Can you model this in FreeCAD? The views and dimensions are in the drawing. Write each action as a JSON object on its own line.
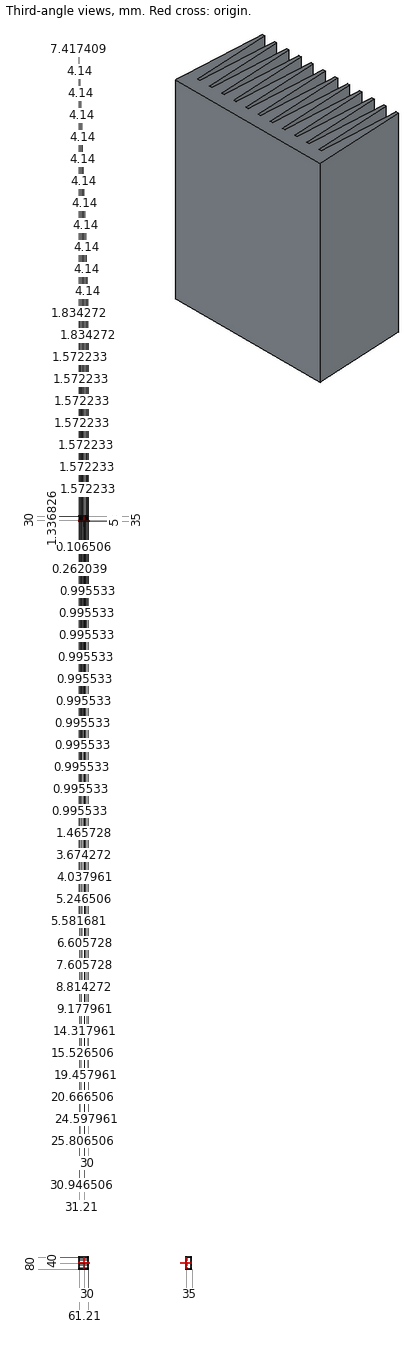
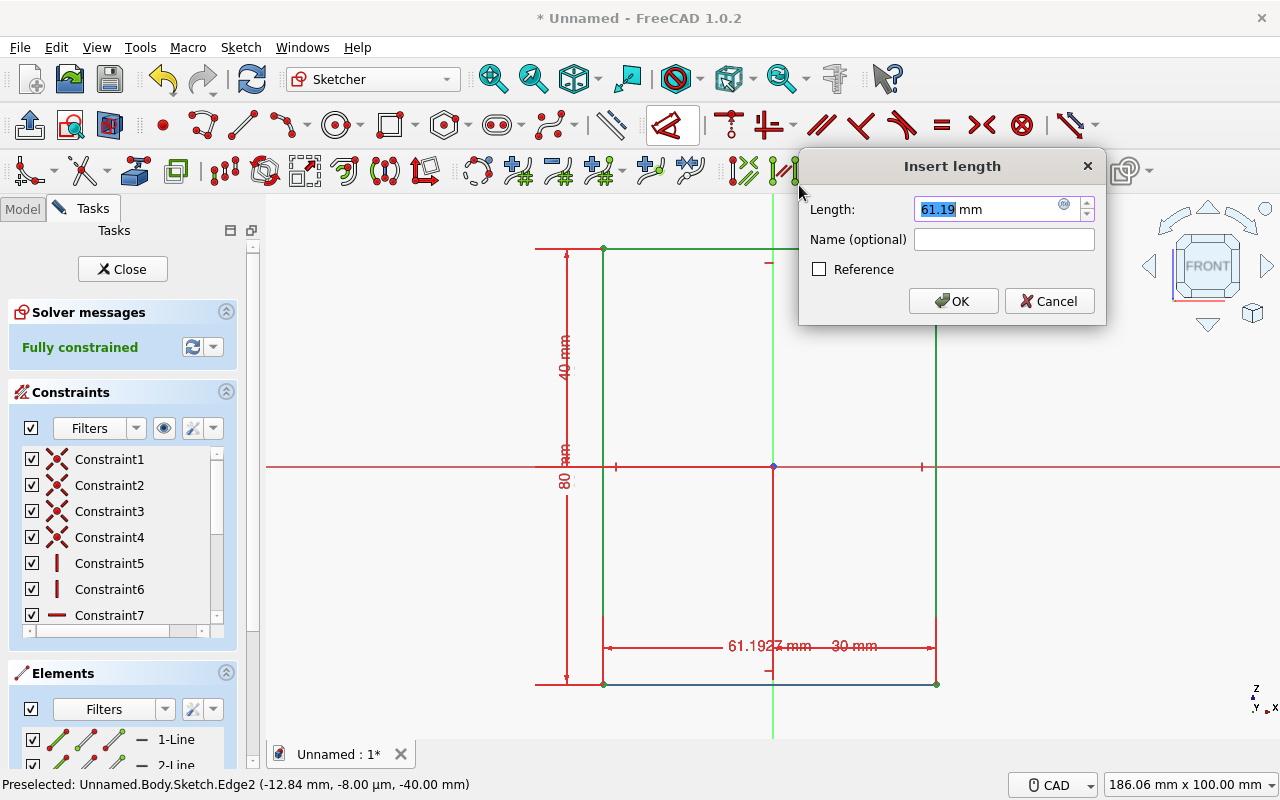
{"action": "type", "text": "61.21"}
{"action": "key", "text": "Return"}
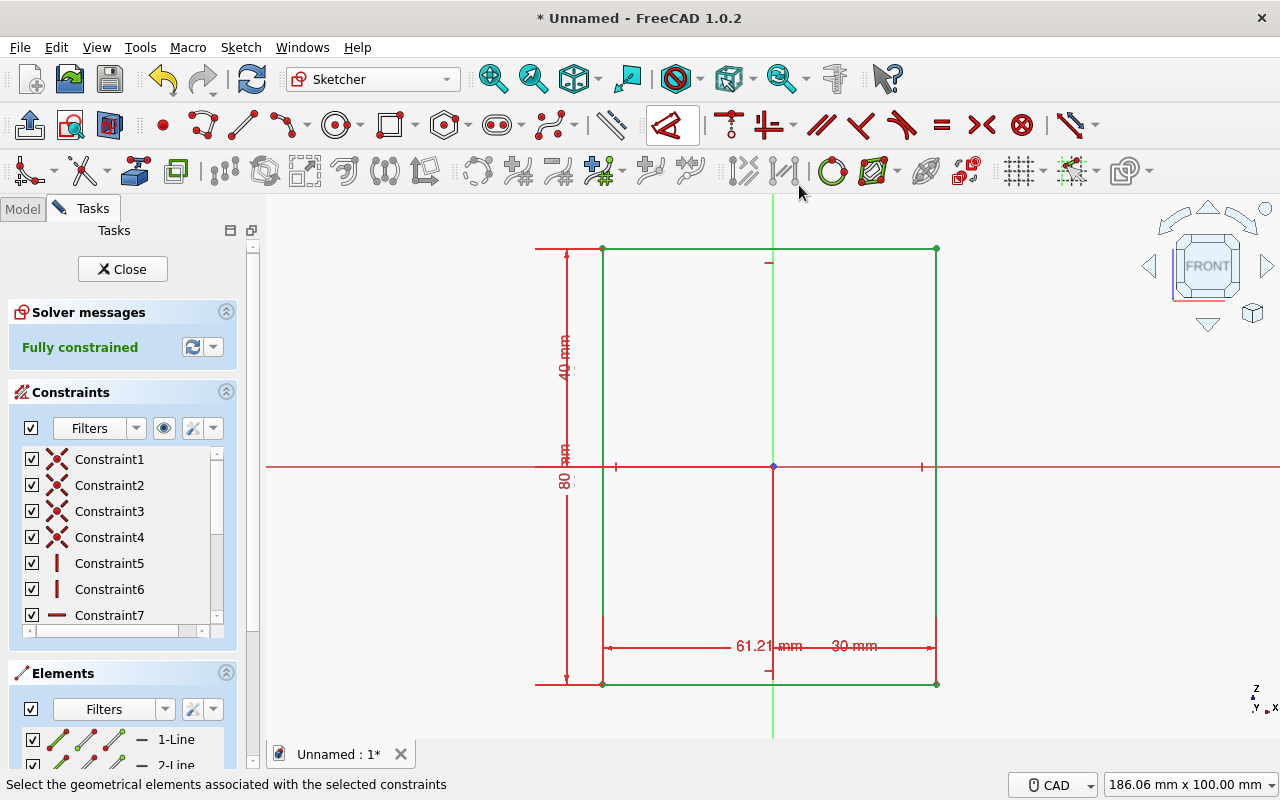
{"action": "left_click", "coordinate": [123, 269]}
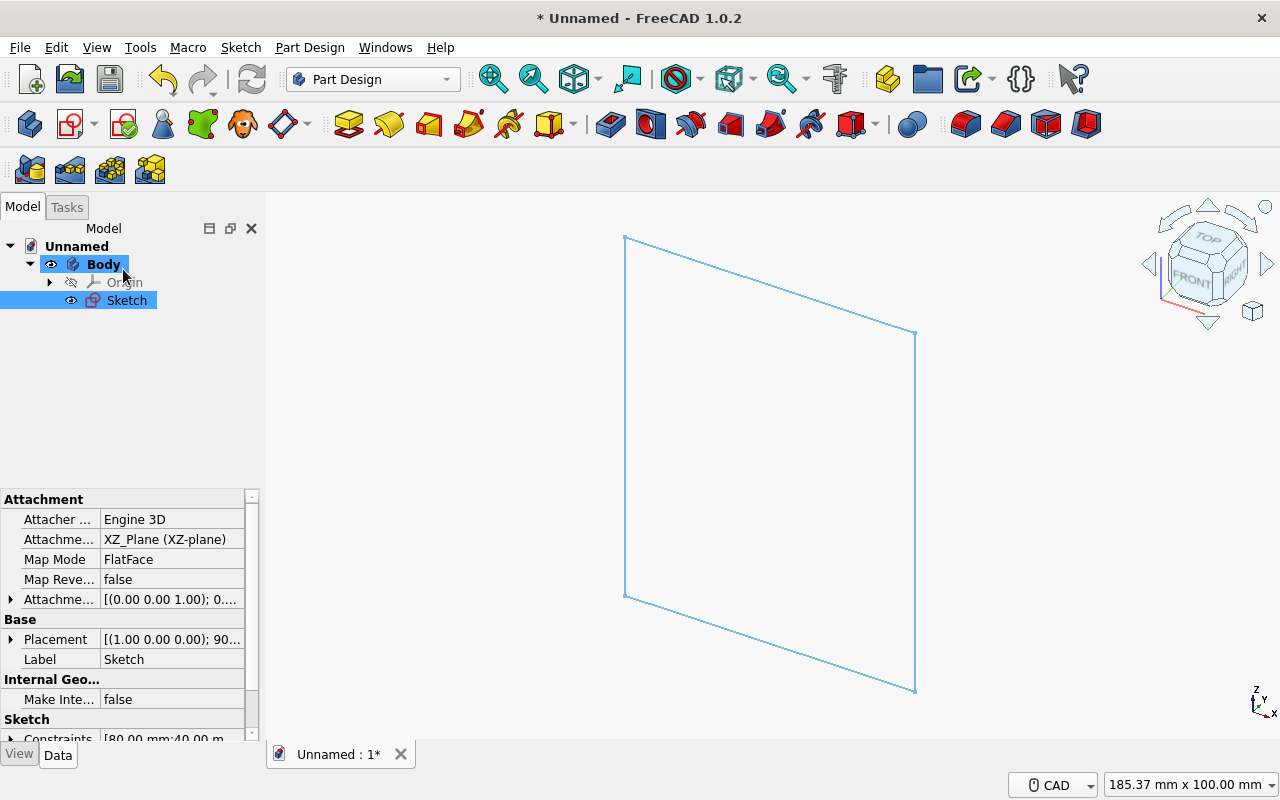
{"action": "left_click", "coordinate": [350, 124]}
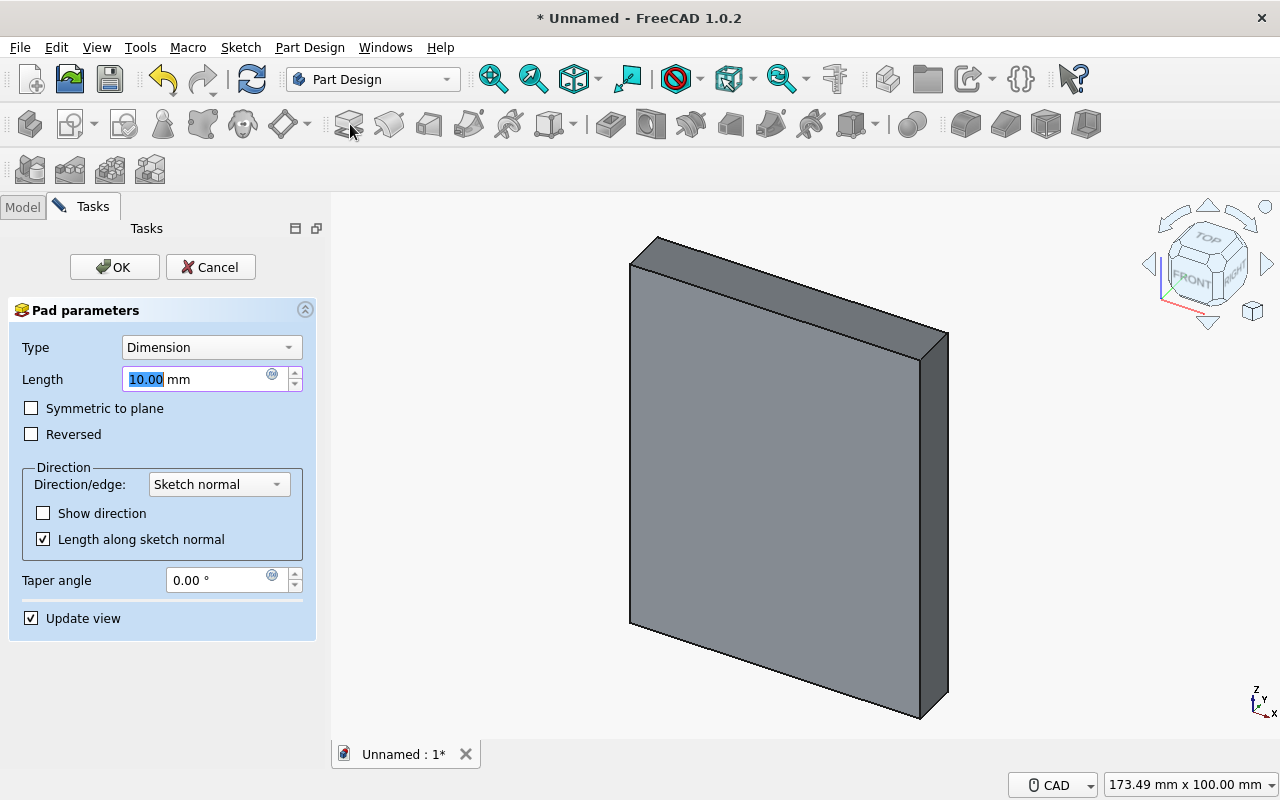
{"action": "type", "text": "35"}
{"action": "key", "text": "Tab"}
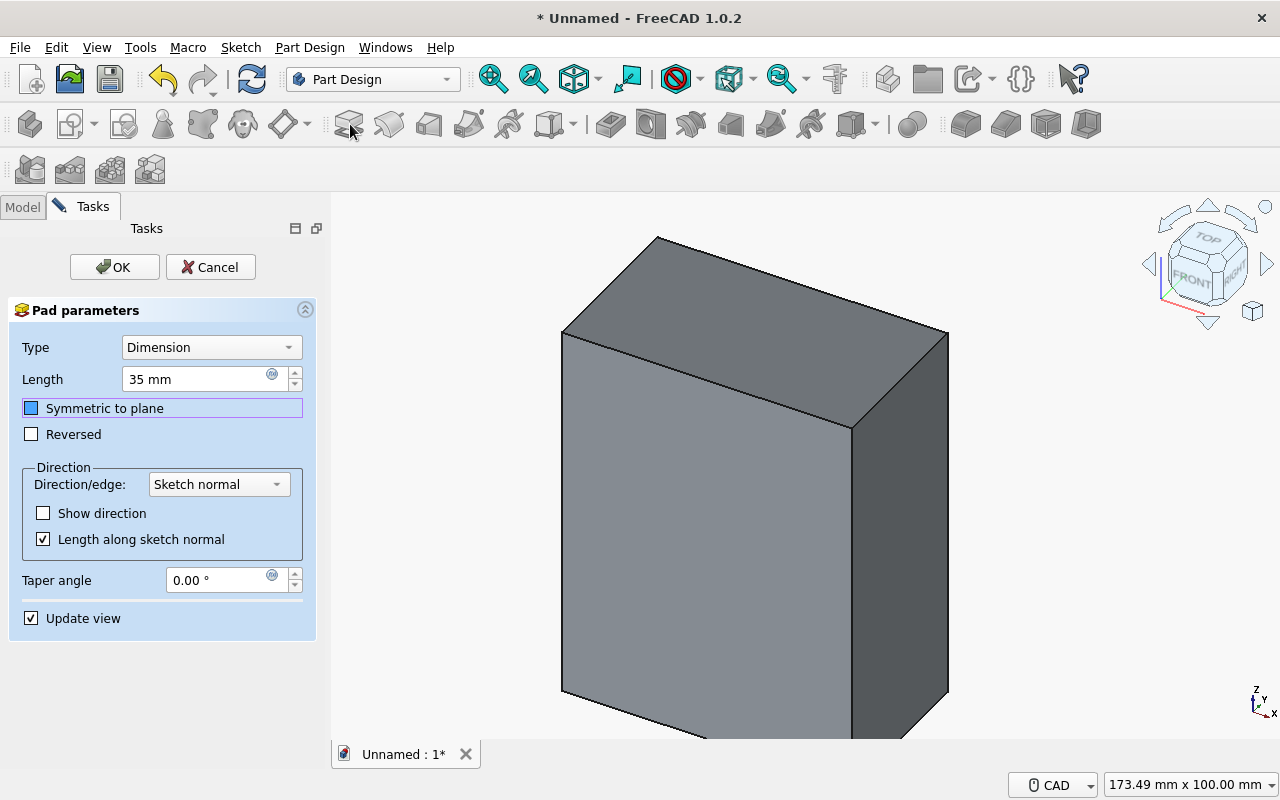
{"action": "left_click", "coordinate": [30, 434]}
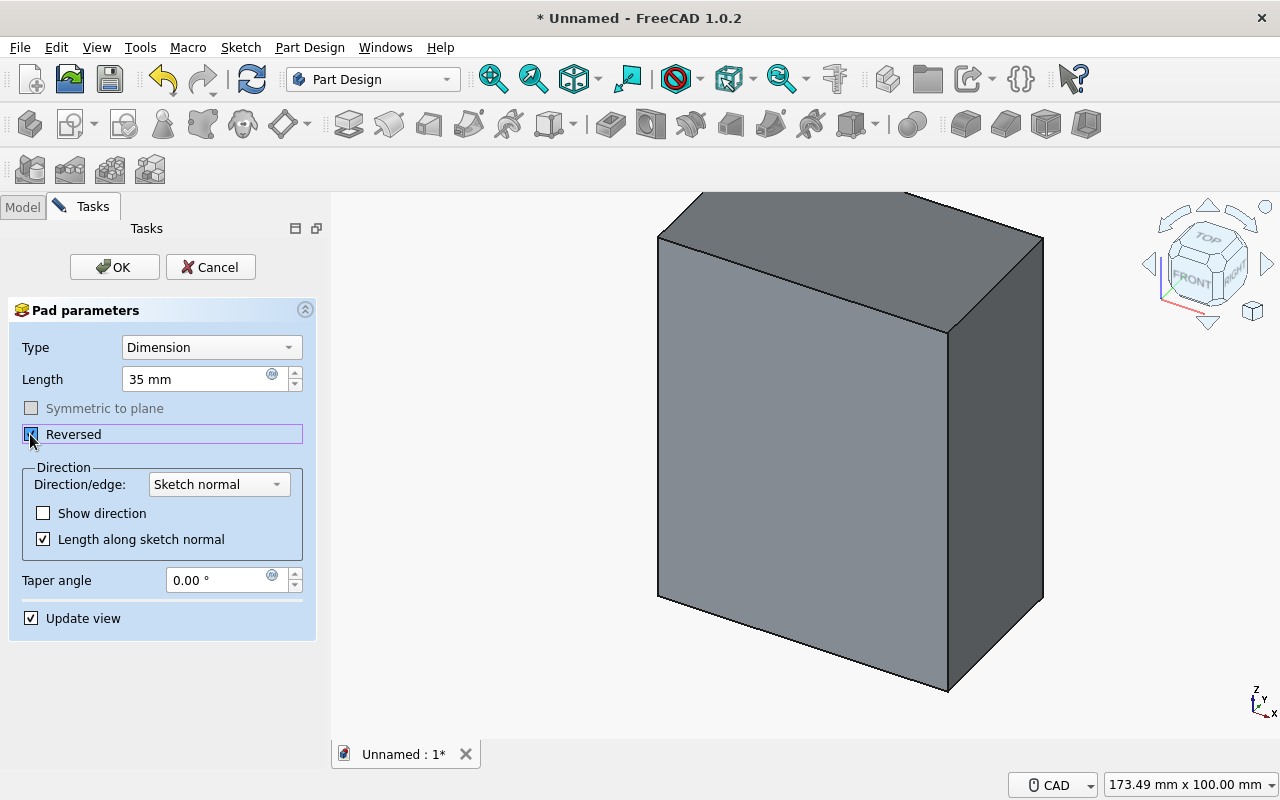
{"action": "left_click", "coordinate": [115, 267]}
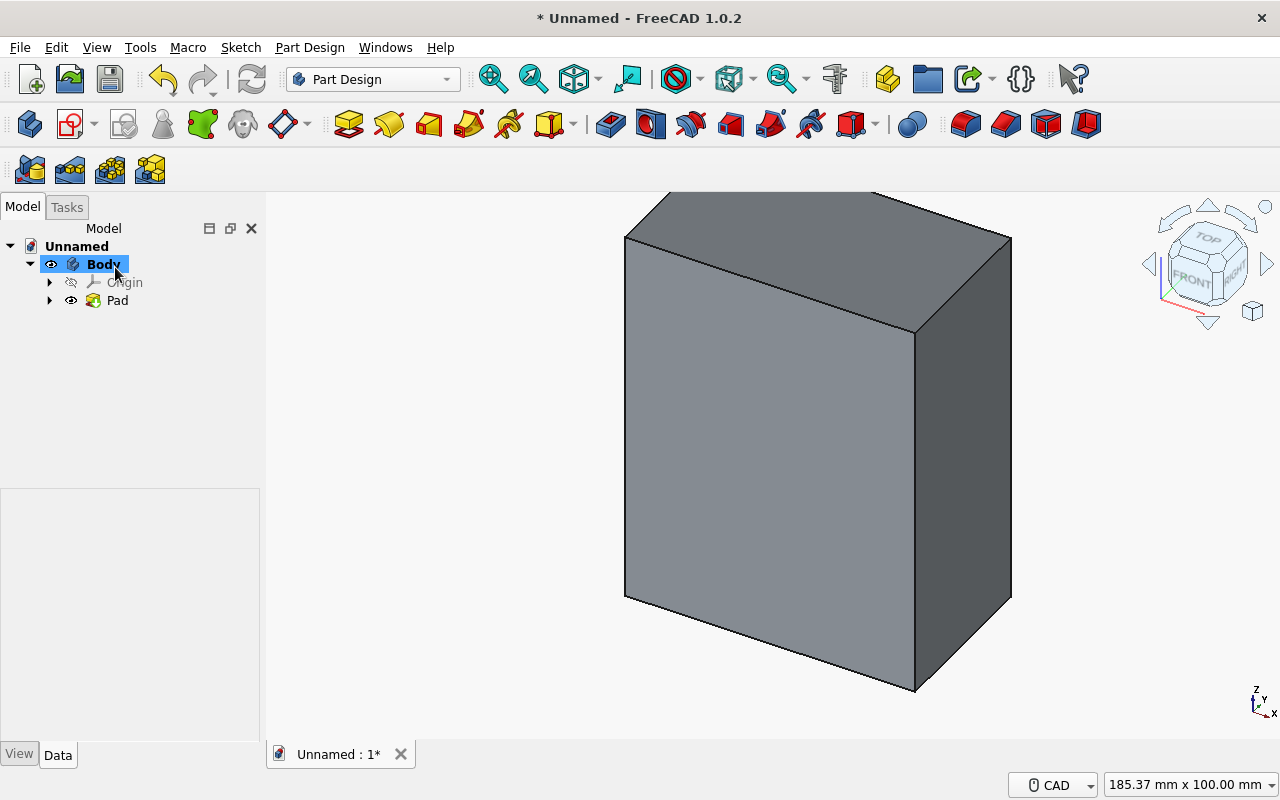
{"action": "left_click", "coordinate": [494, 80]}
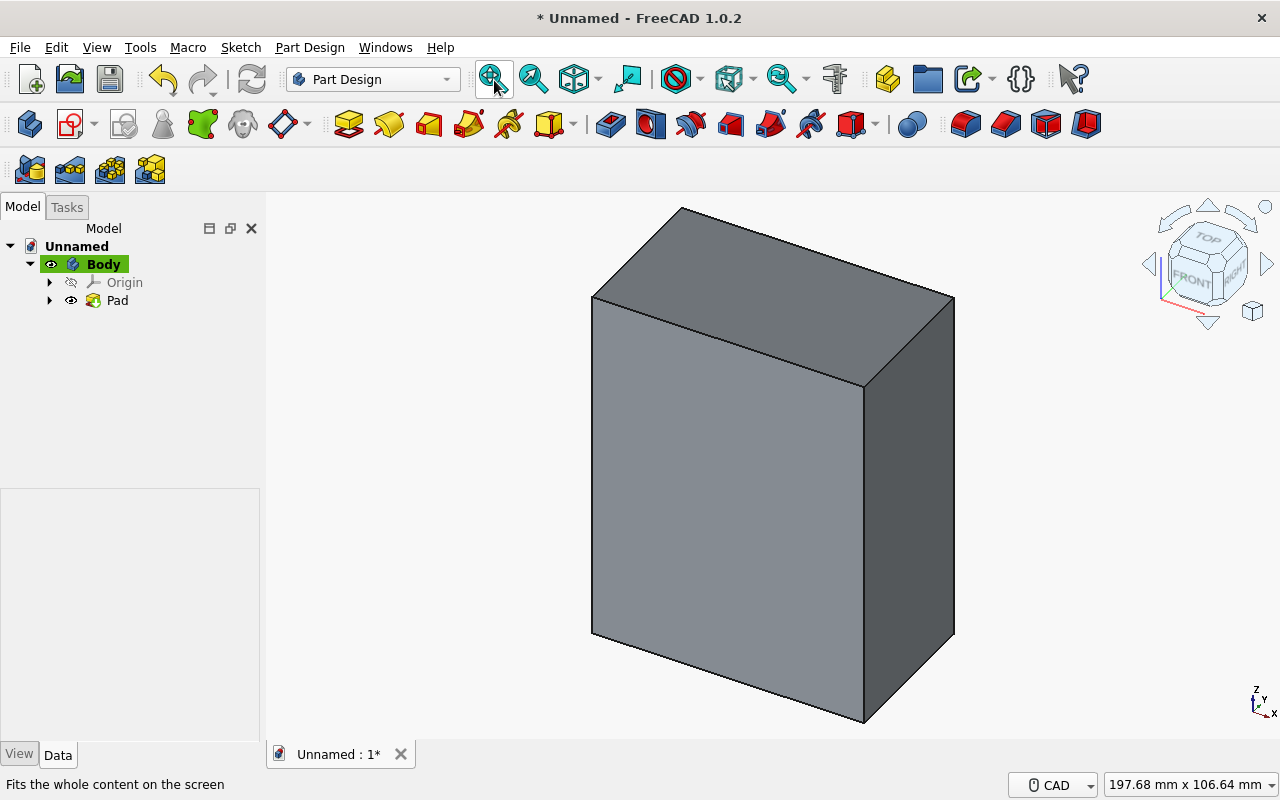
{"action": "left_click", "coordinate": [812, 309]}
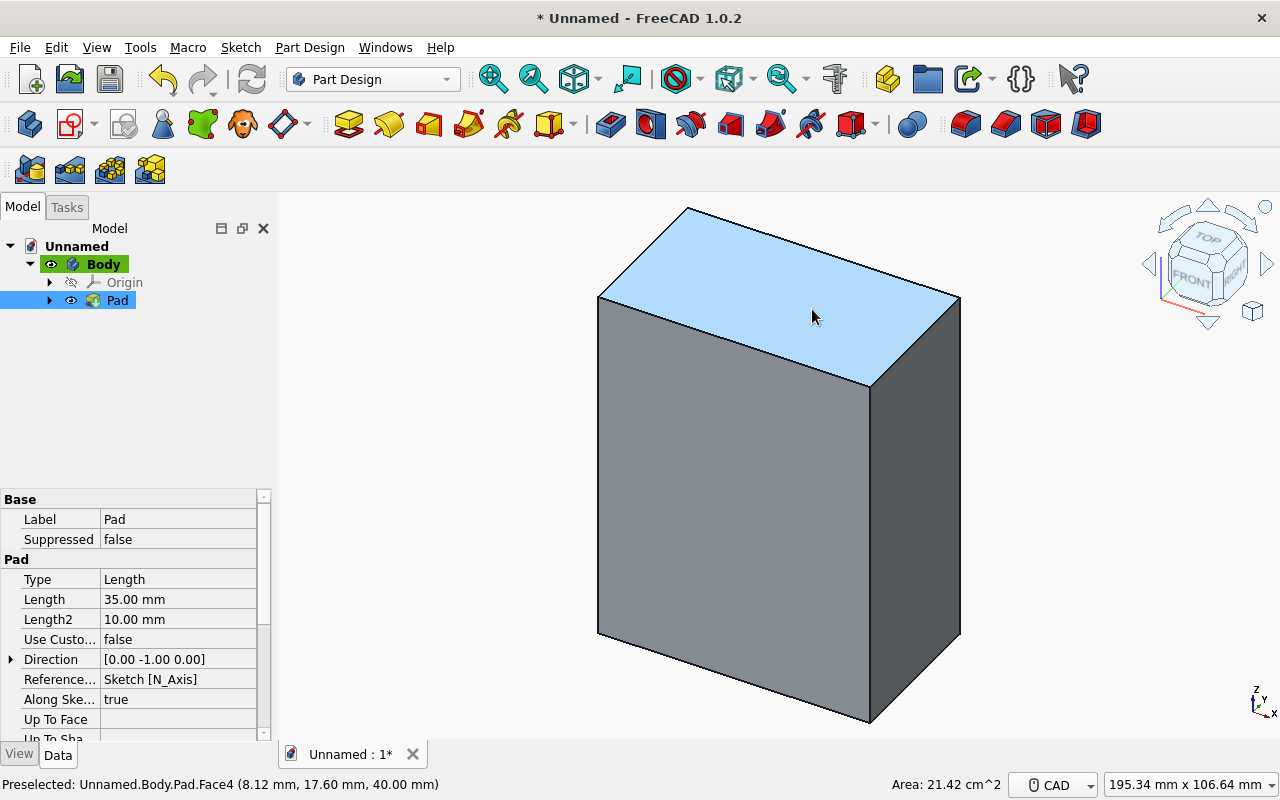
{"action": "left_click", "coordinate": [70, 124]}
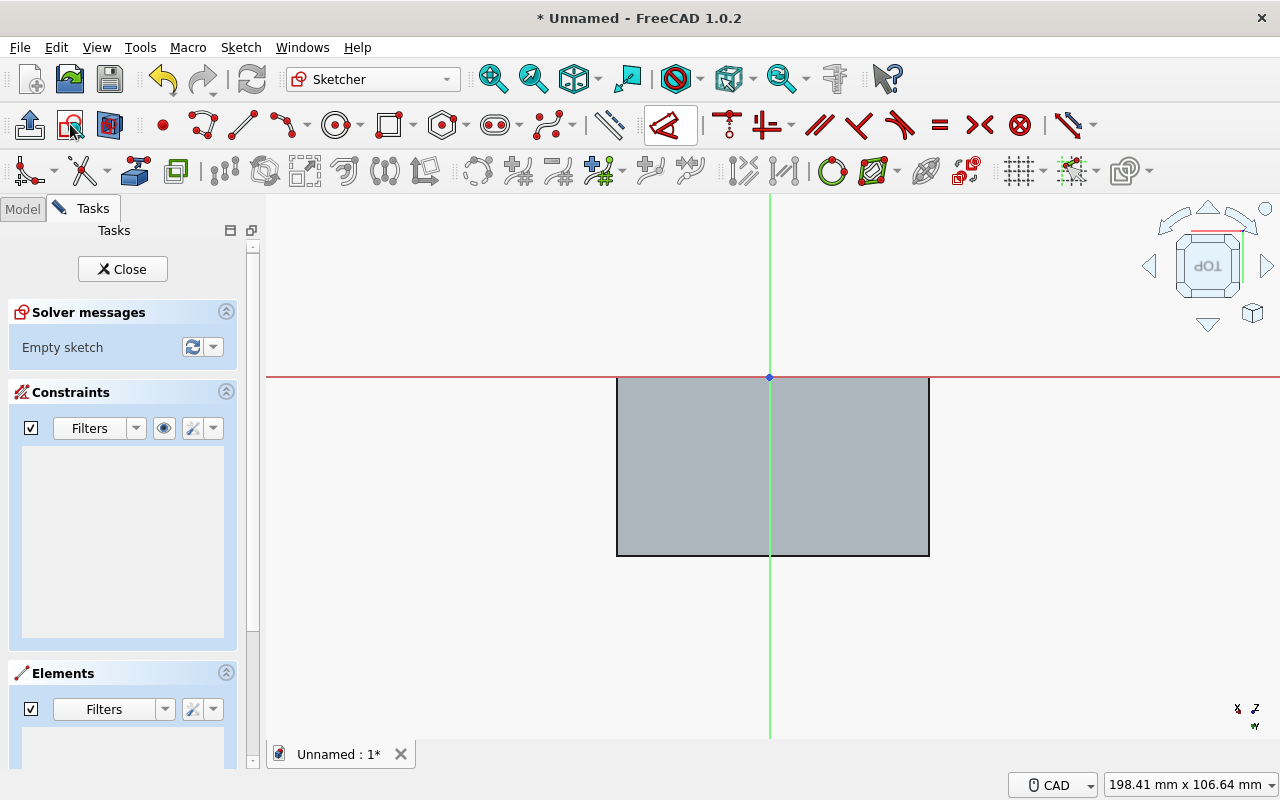
{"action": "scroll", "coordinate": [856, 466], "scroll_direction": "up", "scroll_amount": 3}